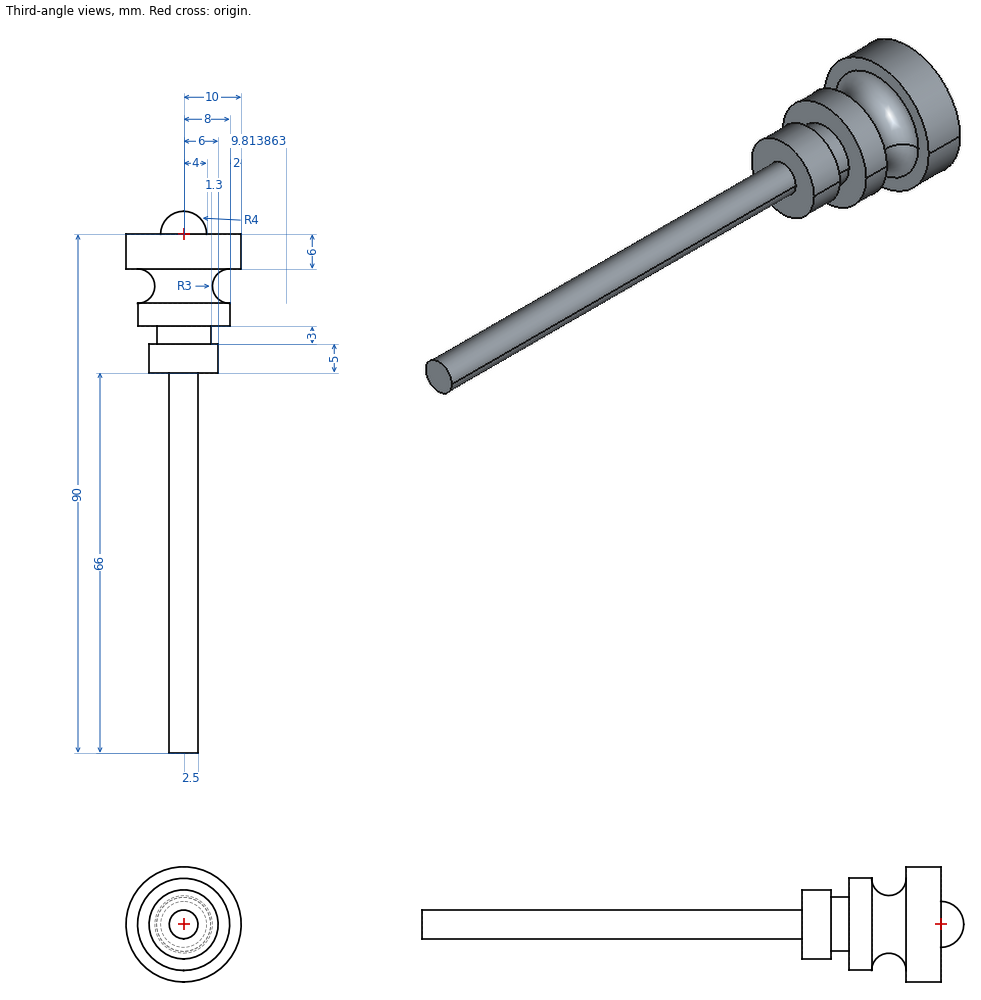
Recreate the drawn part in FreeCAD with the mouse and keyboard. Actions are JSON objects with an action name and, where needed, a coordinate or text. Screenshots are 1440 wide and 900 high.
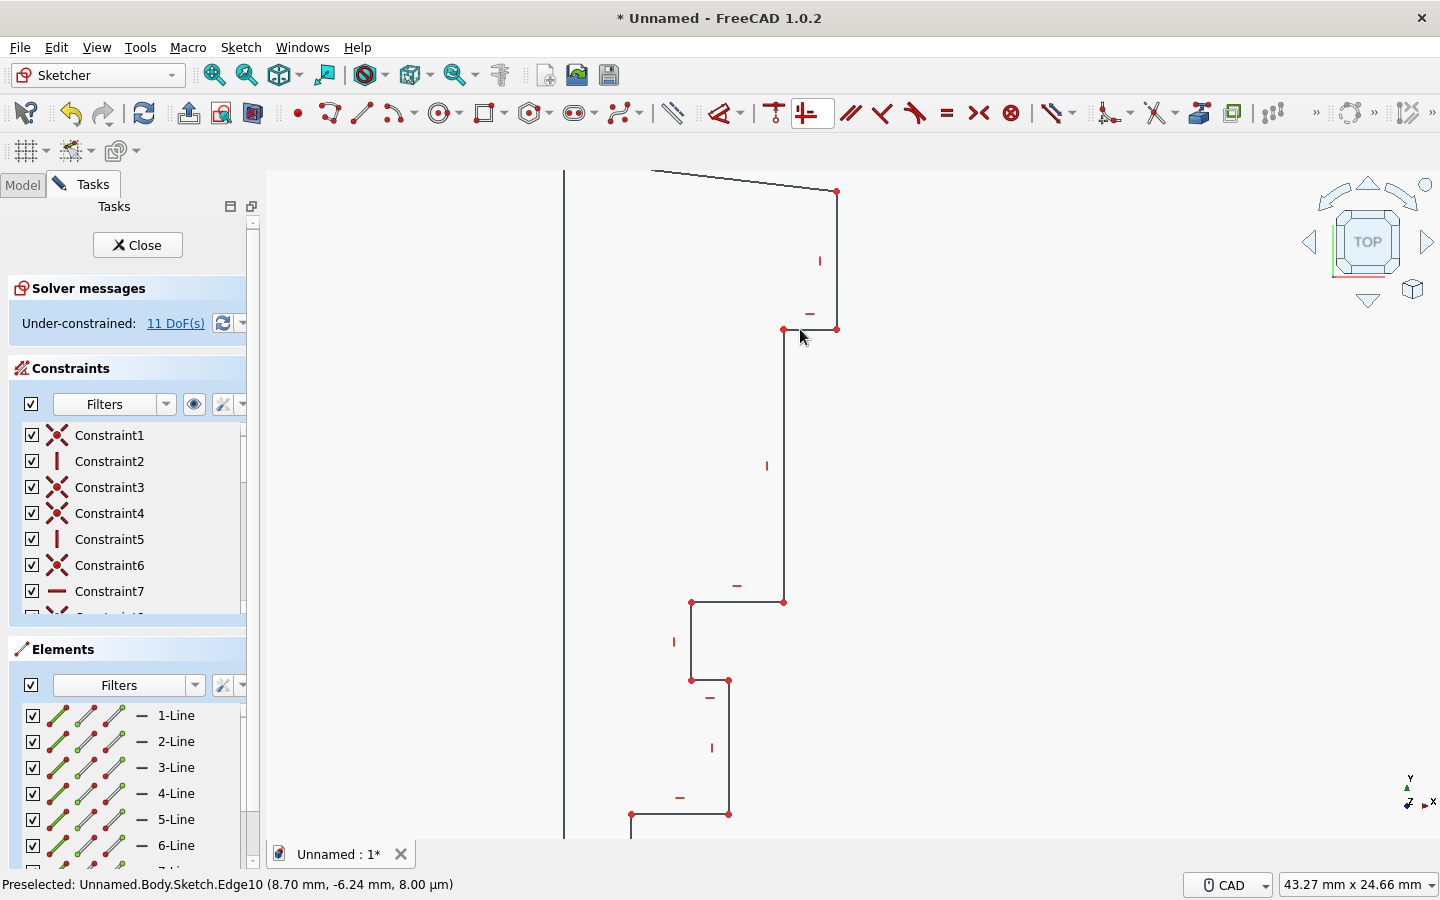
{"action": "scroll", "coordinate": [801, 331], "scroll_direction": "down", "scroll_amount": 9}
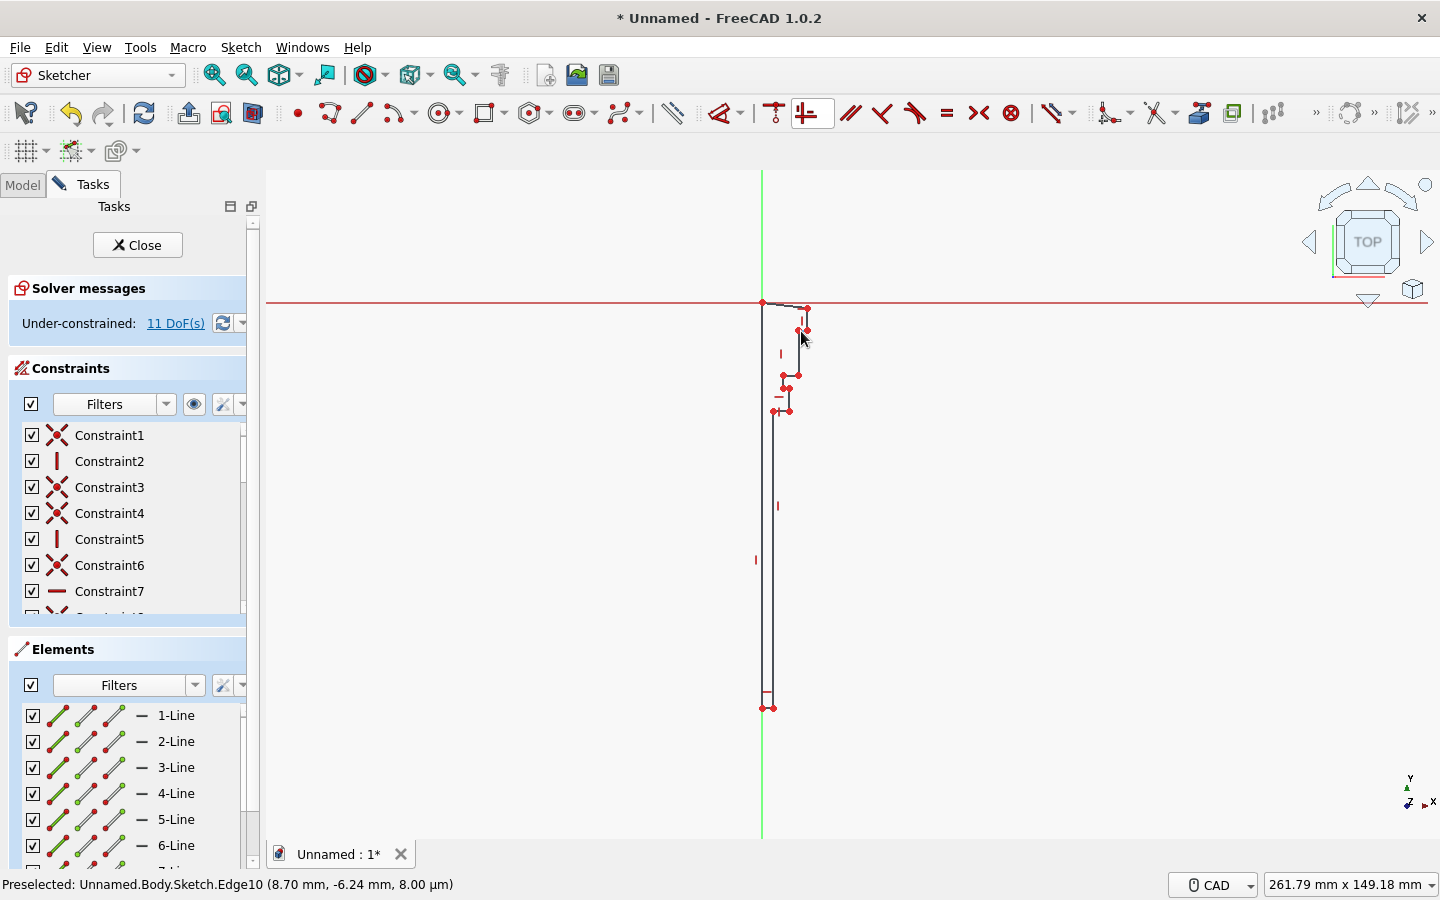
{"action": "scroll", "coordinate": [794, 307], "scroll_direction": "up", "scroll_amount": 7}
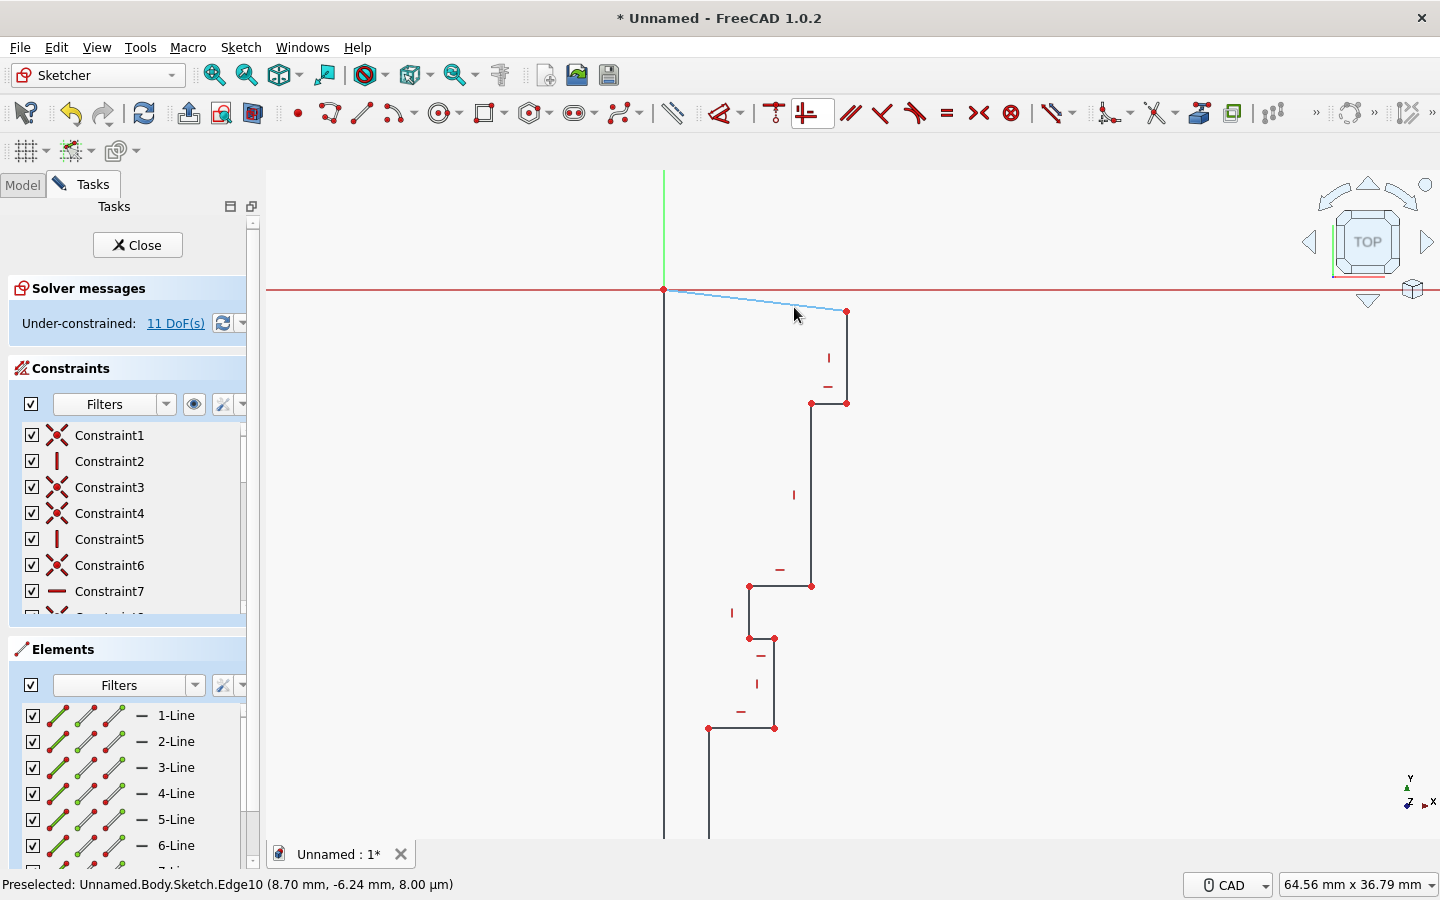
{"action": "left_click", "coordinate": [792, 305]}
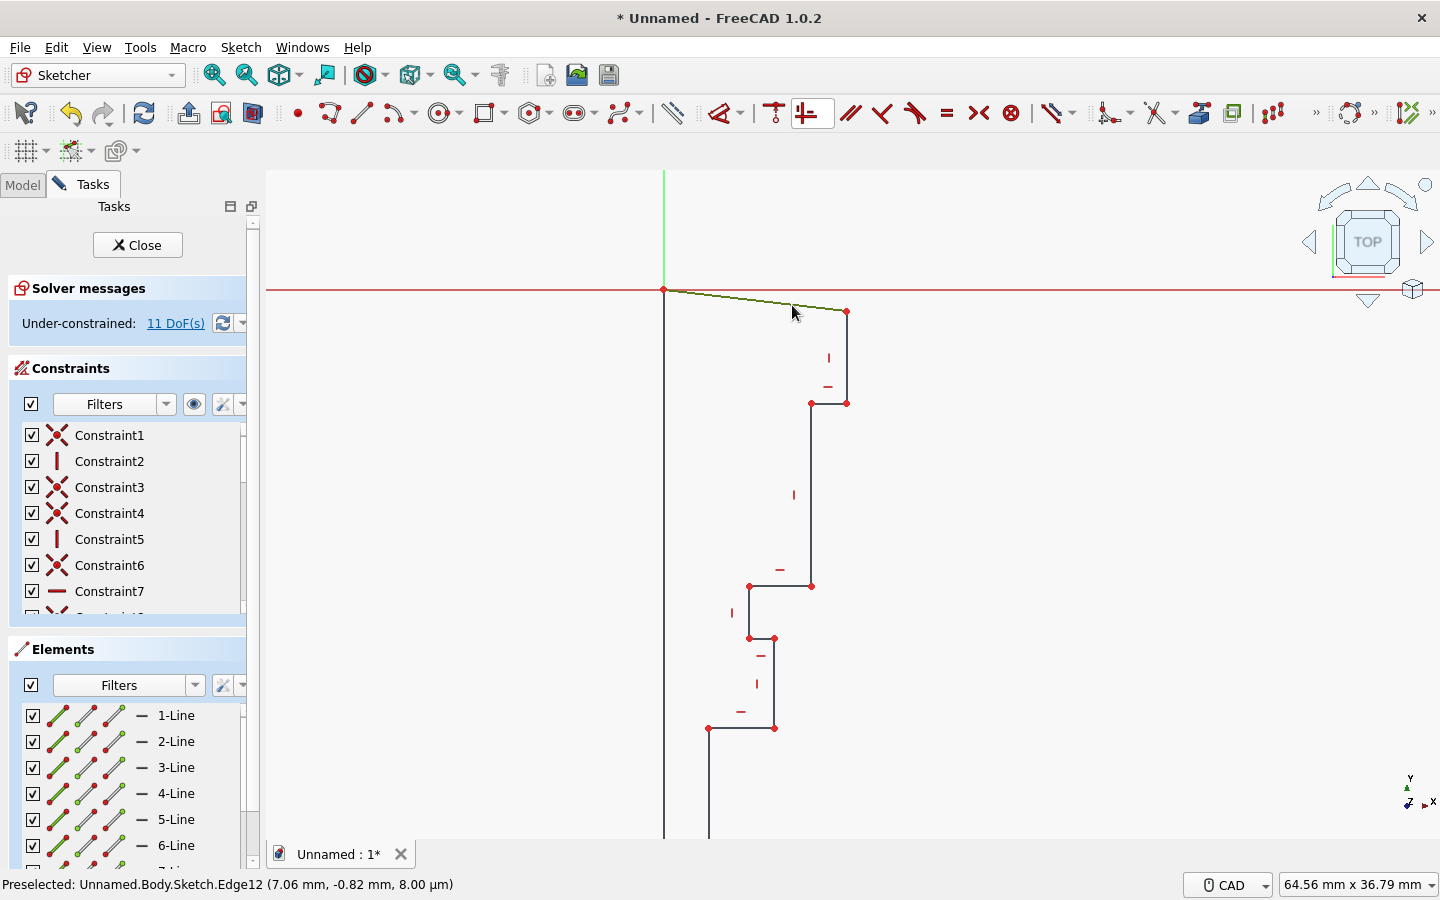
{"action": "left_click", "coordinate": [828, 114]}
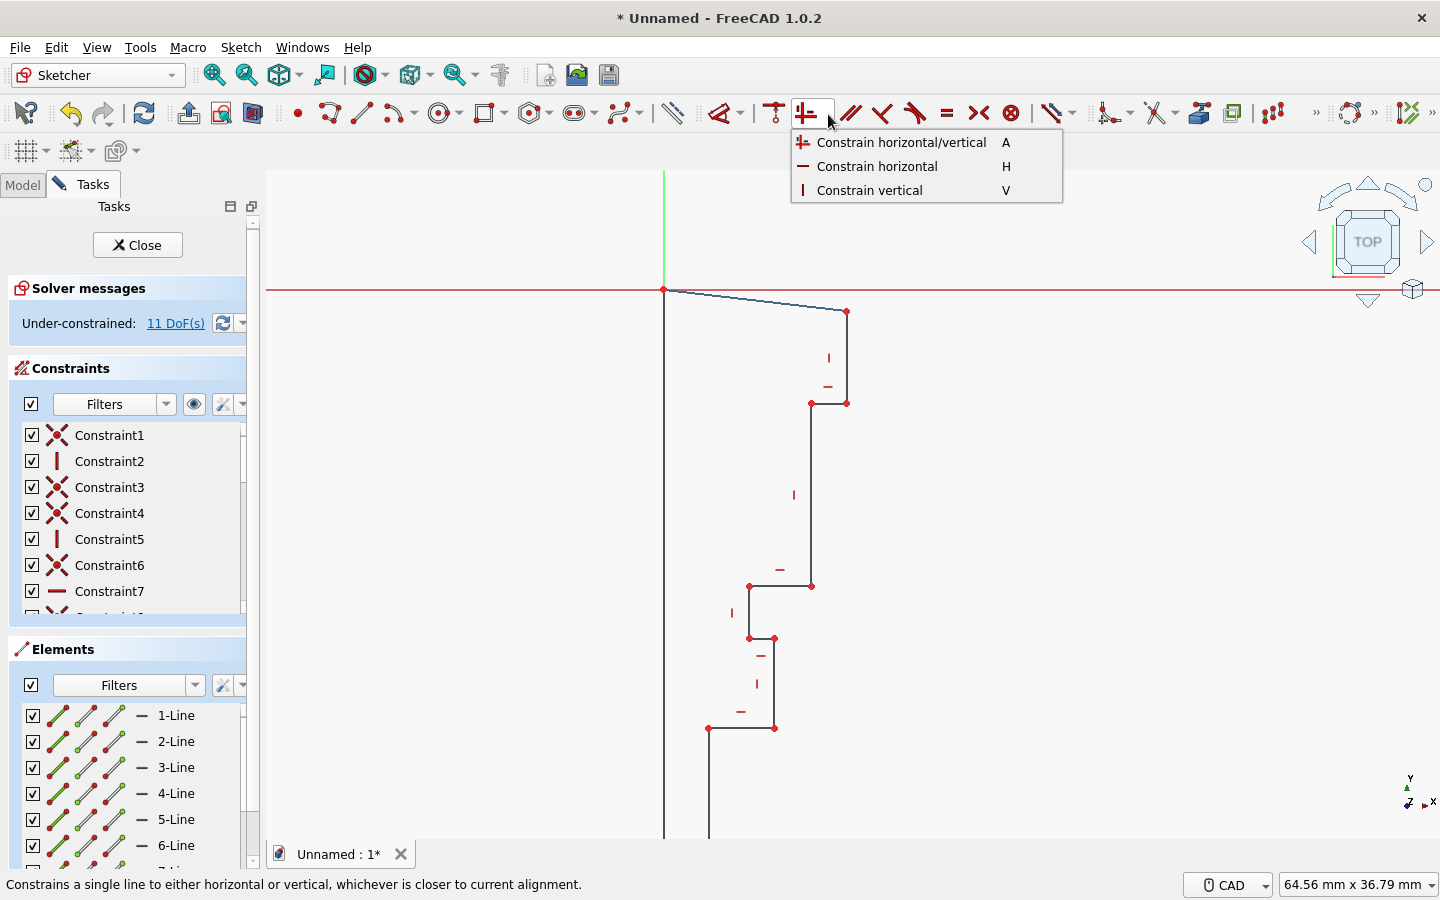
{"action": "left_click", "coordinate": [927, 166]}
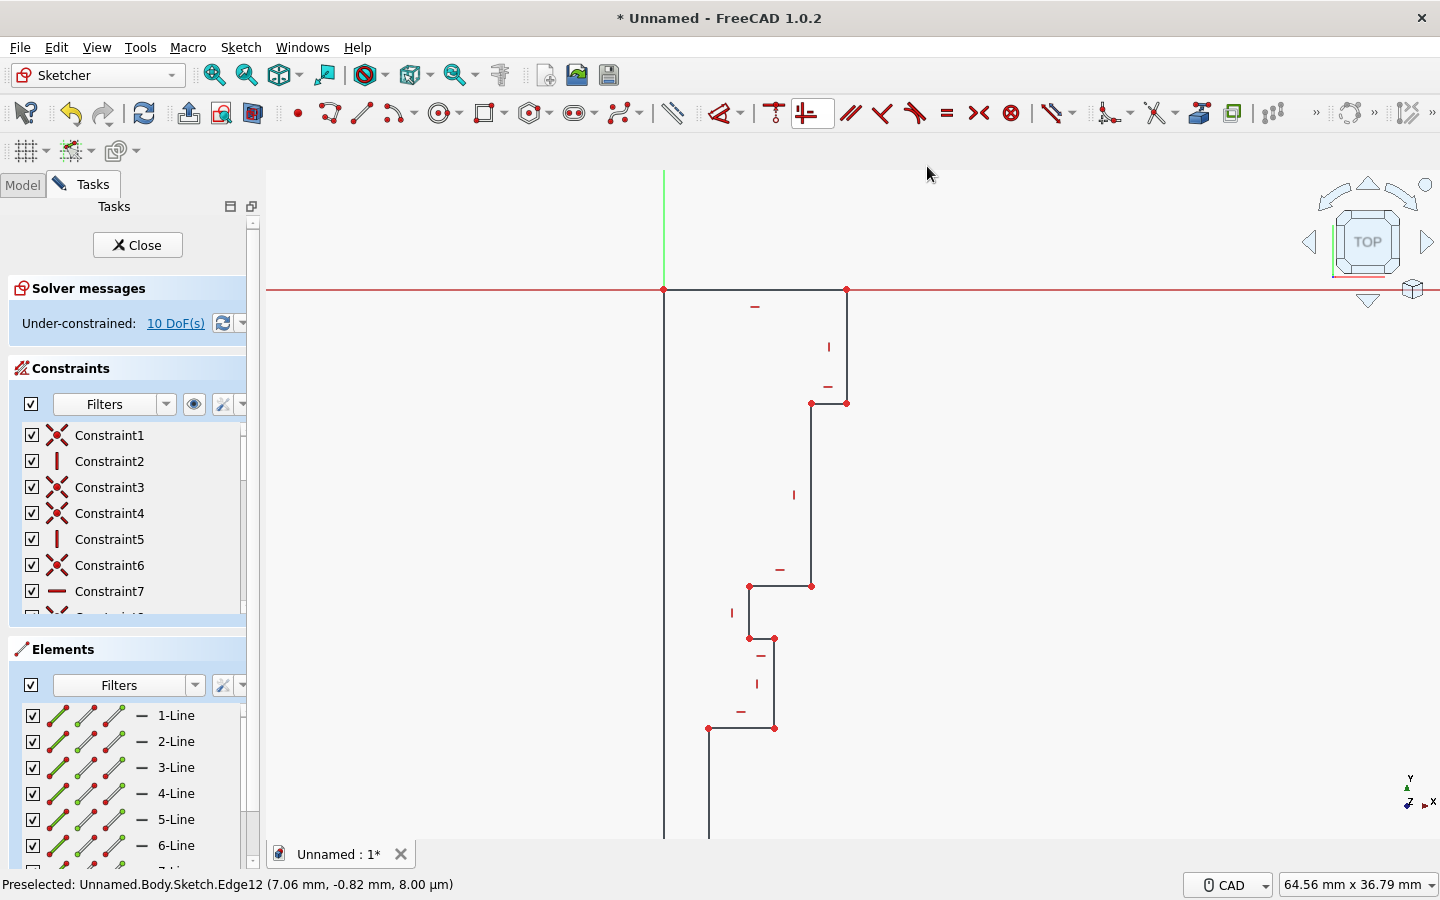
{"action": "left_click", "coordinate": [774, 702]}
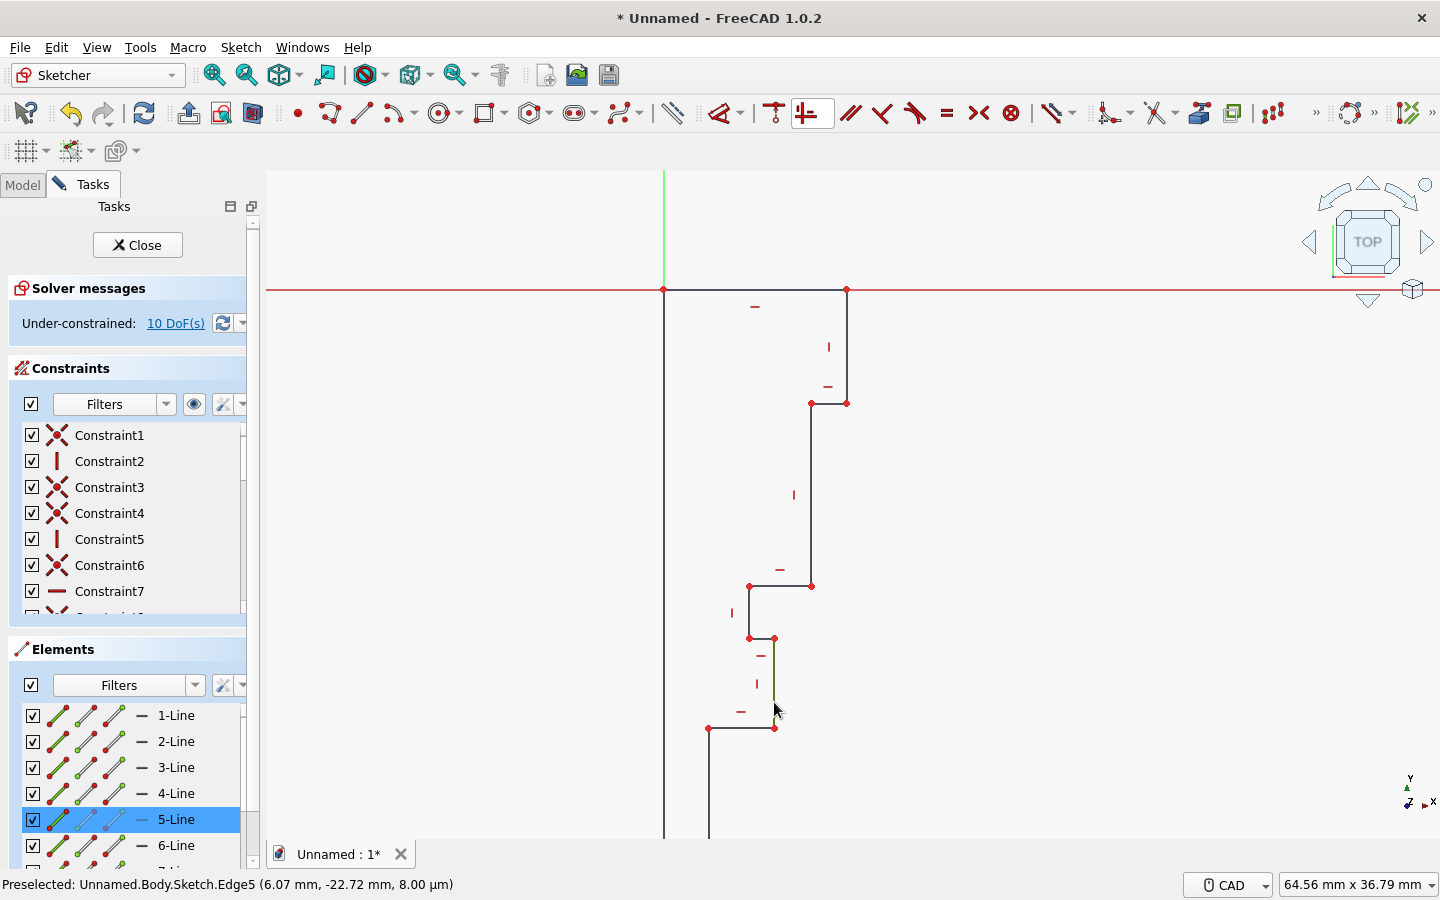
{"action": "key", "text": "i"}